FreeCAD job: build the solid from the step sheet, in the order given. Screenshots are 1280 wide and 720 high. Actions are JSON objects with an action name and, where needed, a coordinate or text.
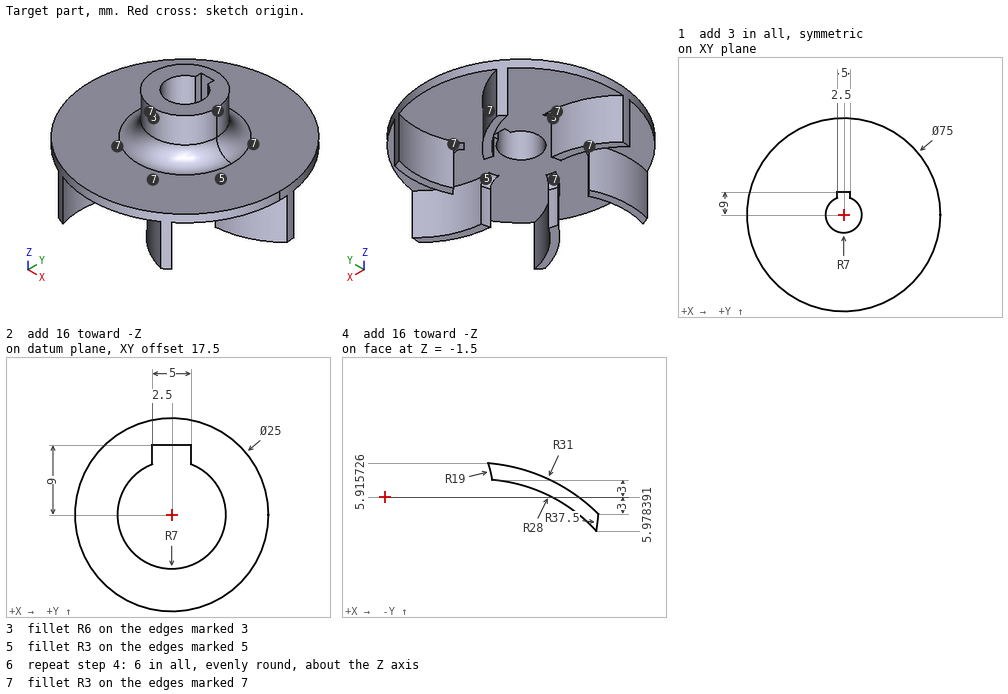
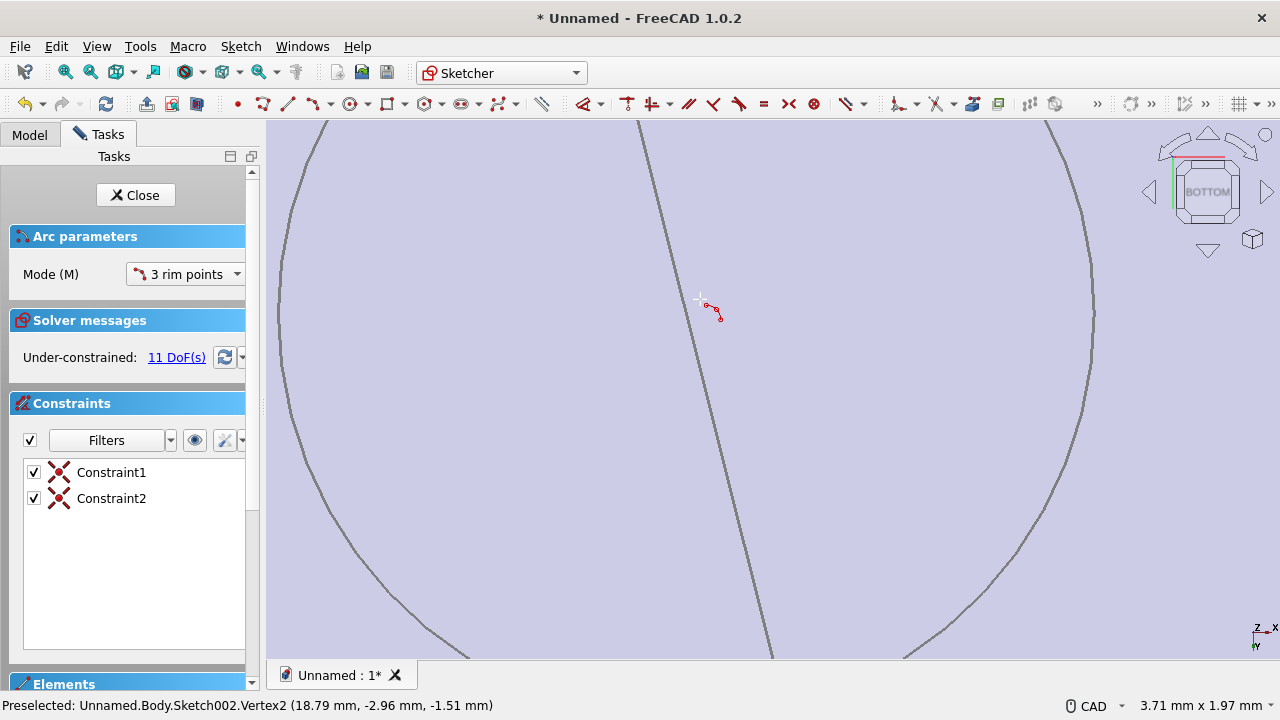
{"action": "left_click", "coordinate": [698, 296]}
{"action": "key", "text": "Escape"}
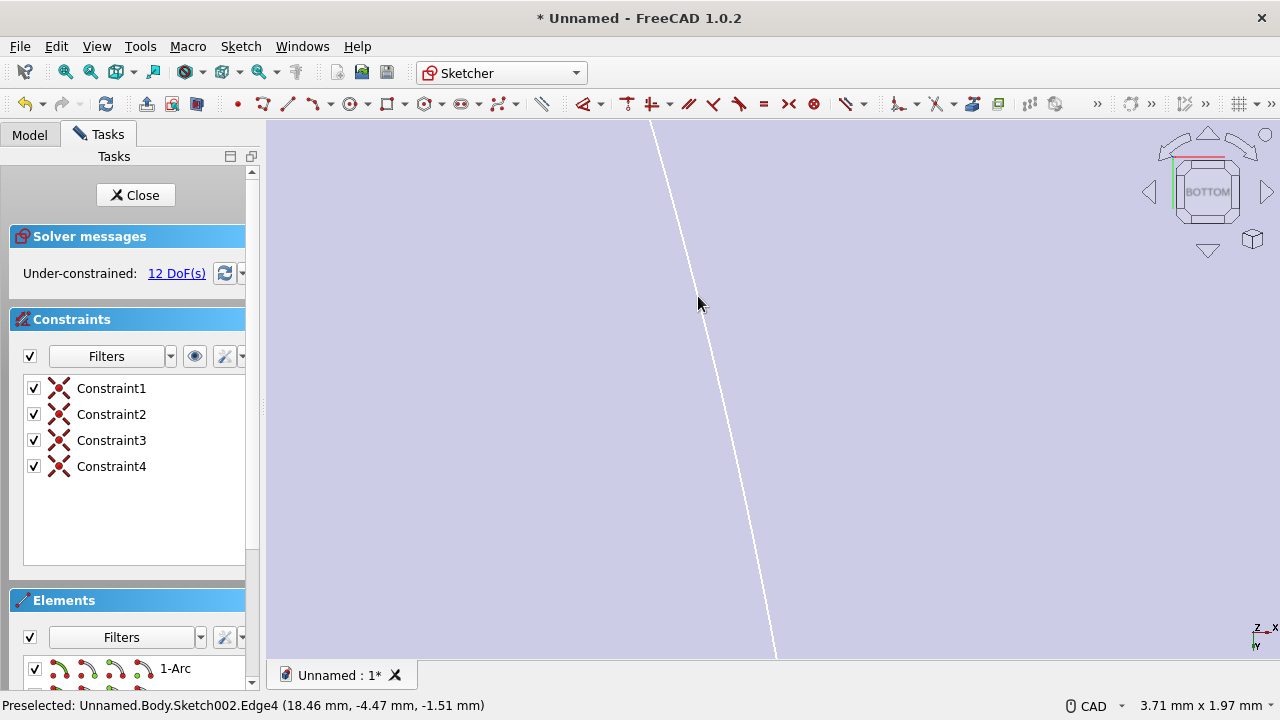
{"action": "scroll", "coordinate": [701, 316], "scroll_direction": "down", "scroll_amount": 14}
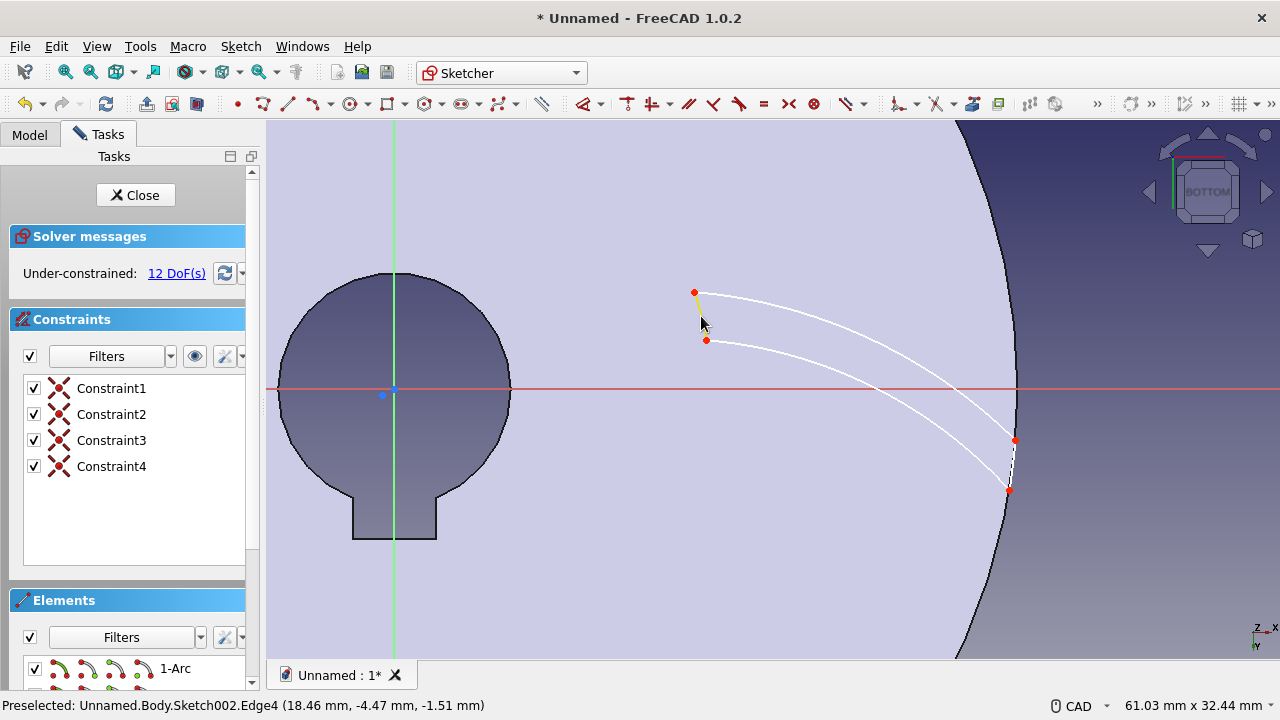
{"action": "left_click", "coordinate": [1012, 475]}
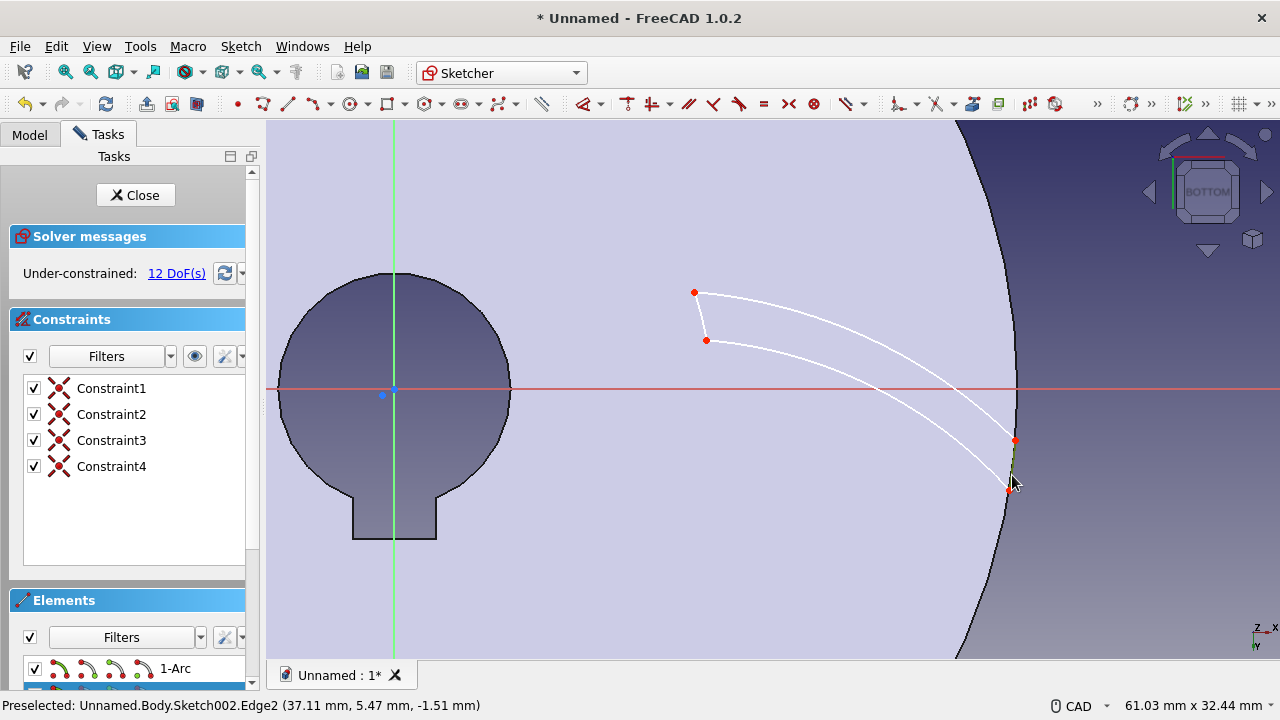
{"action": "left_click", "coordinate": [704, 326]}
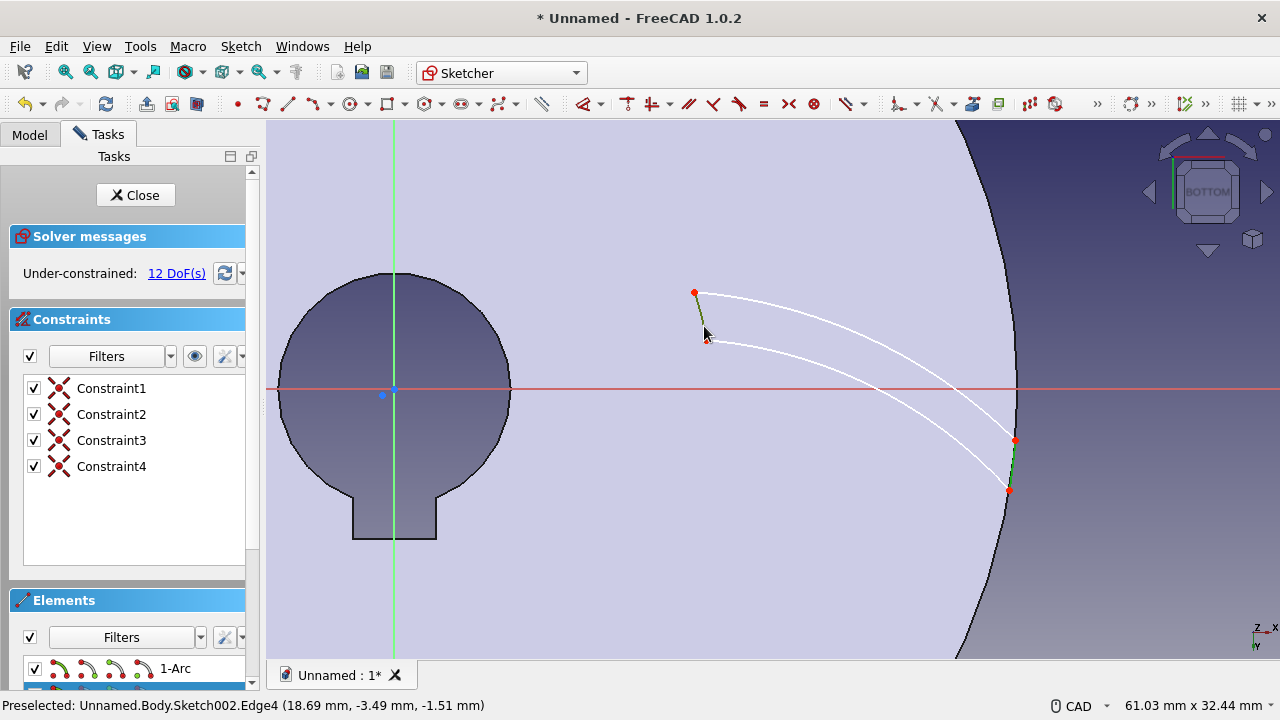
{"action": "left_click", "coordinate": [627, 104]}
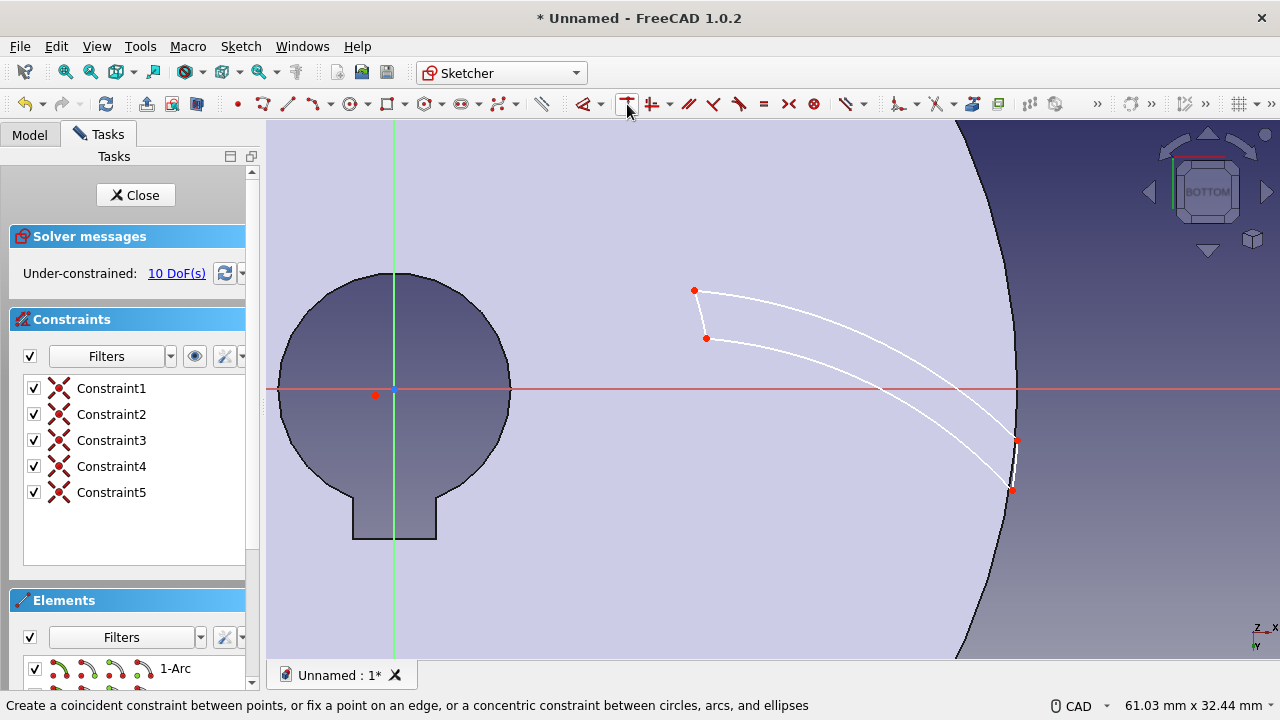
{"action": "left_click_drag", "start_coordinate": [366, 379], "coordinate": [404, 405]}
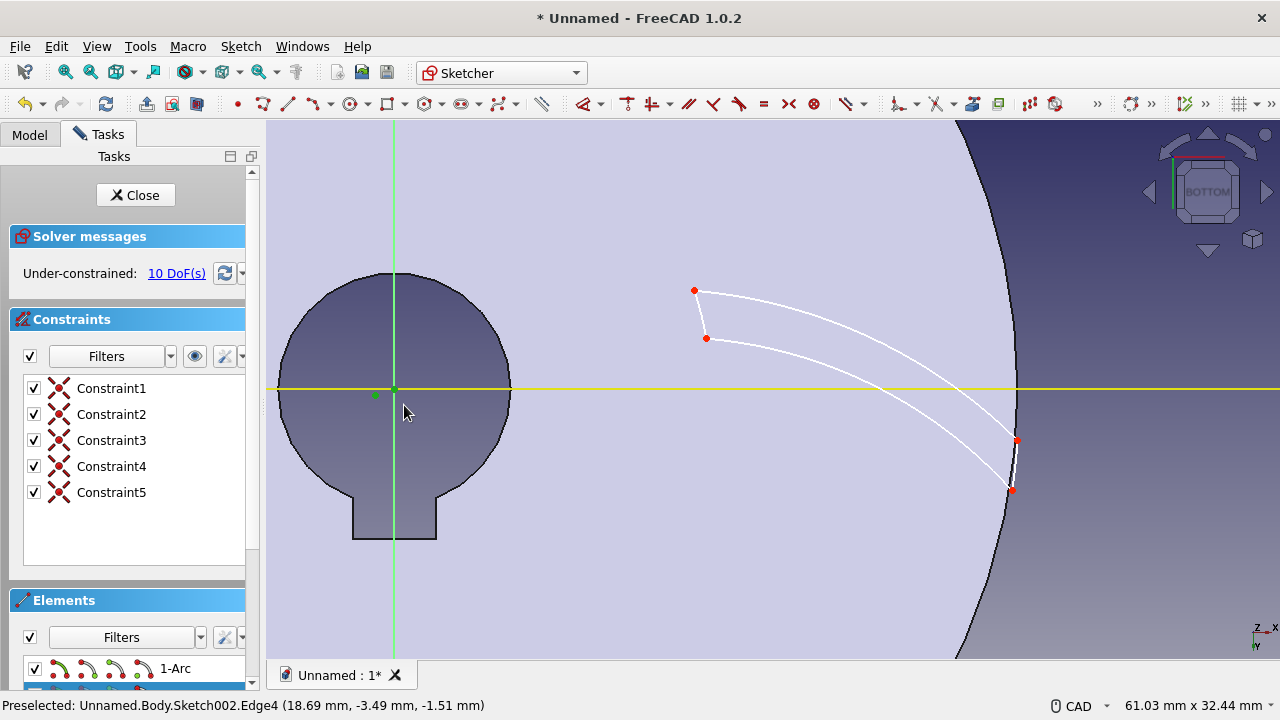
{"action": "key", "text": "c"}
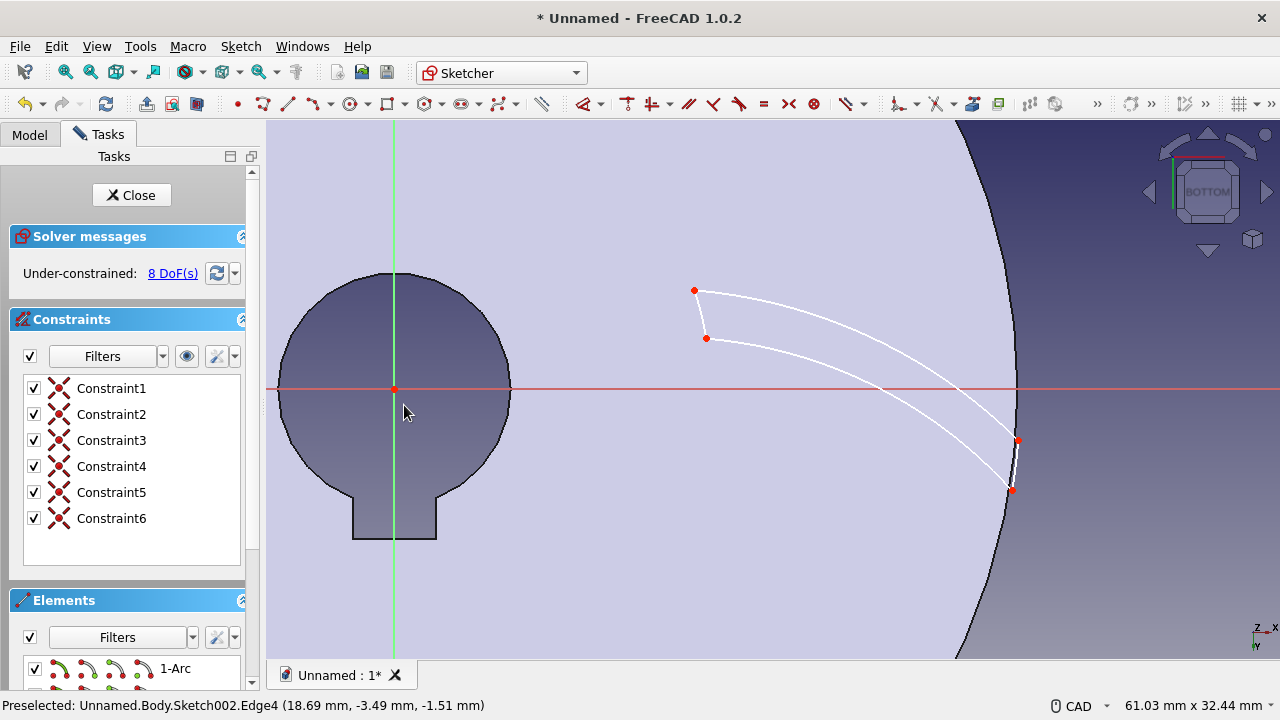
{"action": "left_click", "coordinate": [582, 104]}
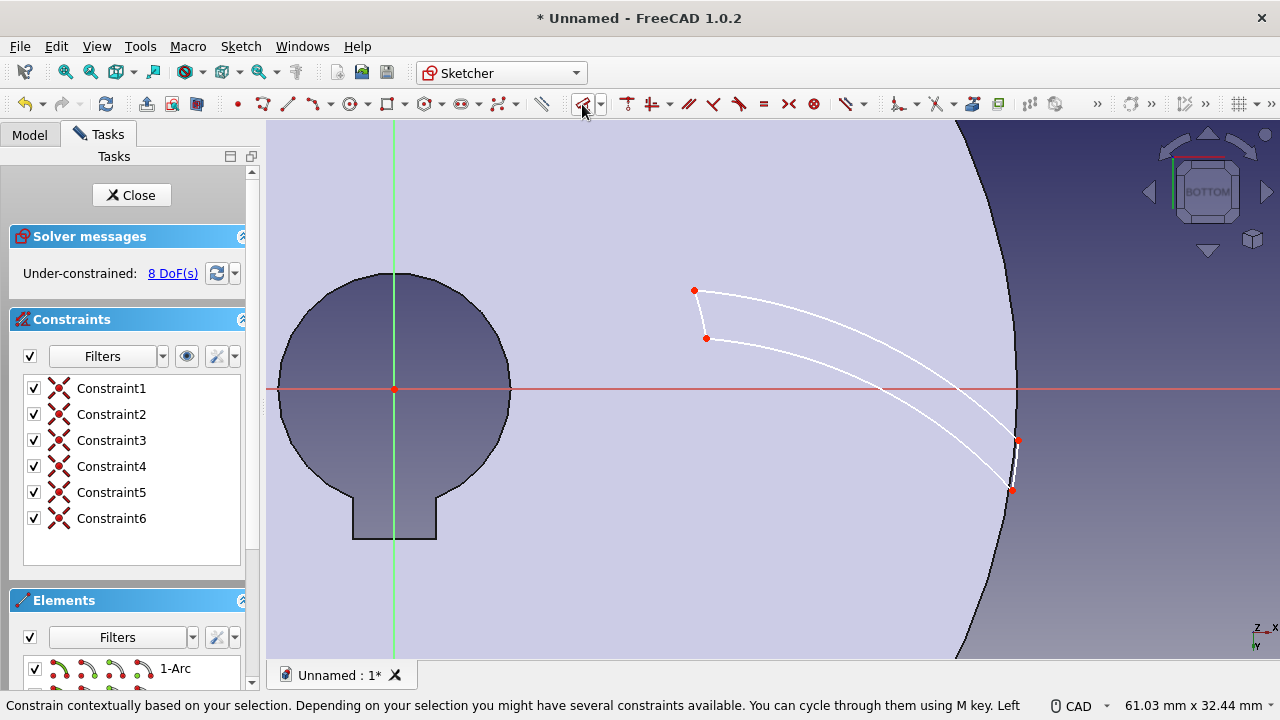
{"action": "left_click", "coordinate": [934, 421]}
{"action": "left_click", "coordinate": [1112, 581]}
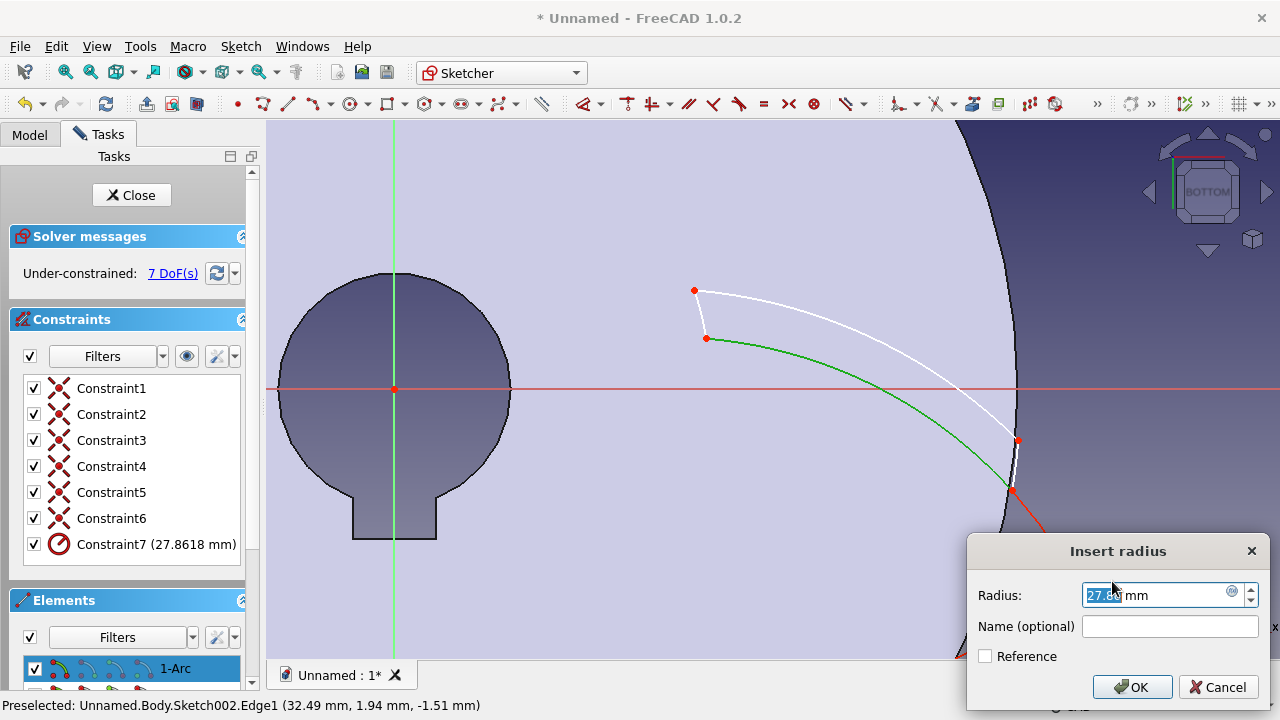
{"action": "type", "text": "28"}
{"action": "key", "text": "Return"}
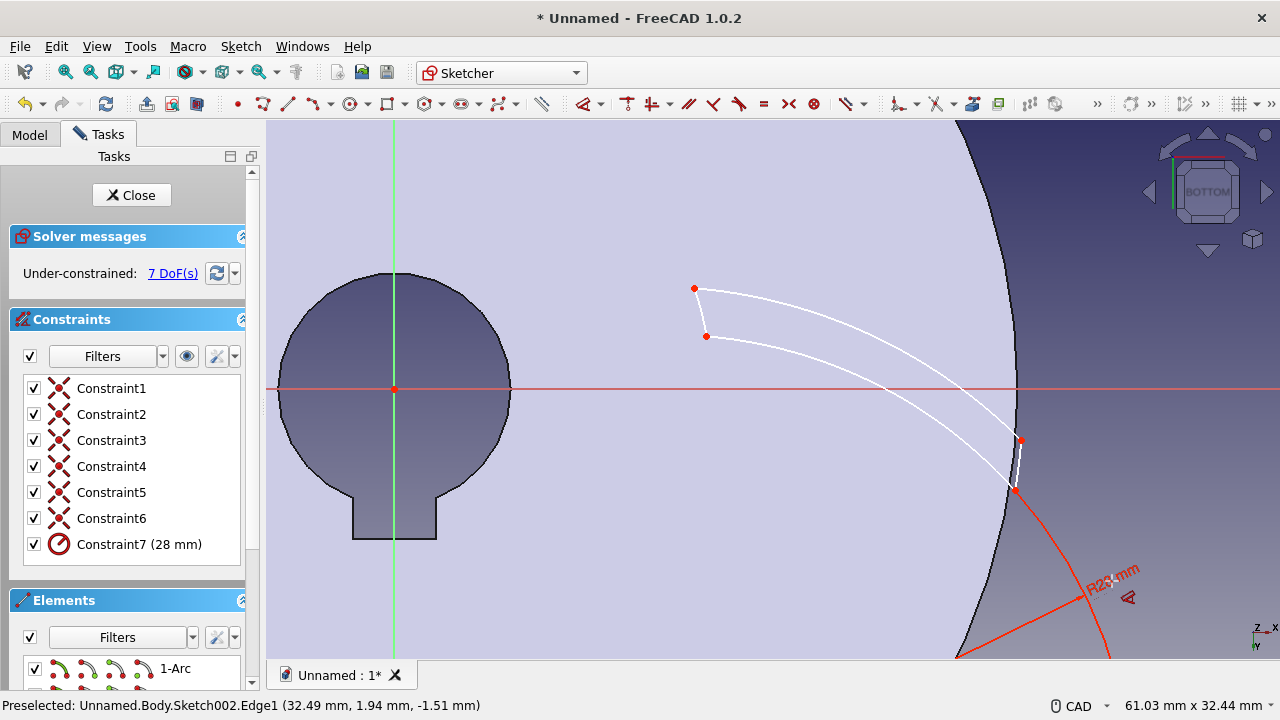
{"action": "left_click", "coordinate": [1017, 476]}
{"action": "left_click", "coordinate": [1049, 480]}